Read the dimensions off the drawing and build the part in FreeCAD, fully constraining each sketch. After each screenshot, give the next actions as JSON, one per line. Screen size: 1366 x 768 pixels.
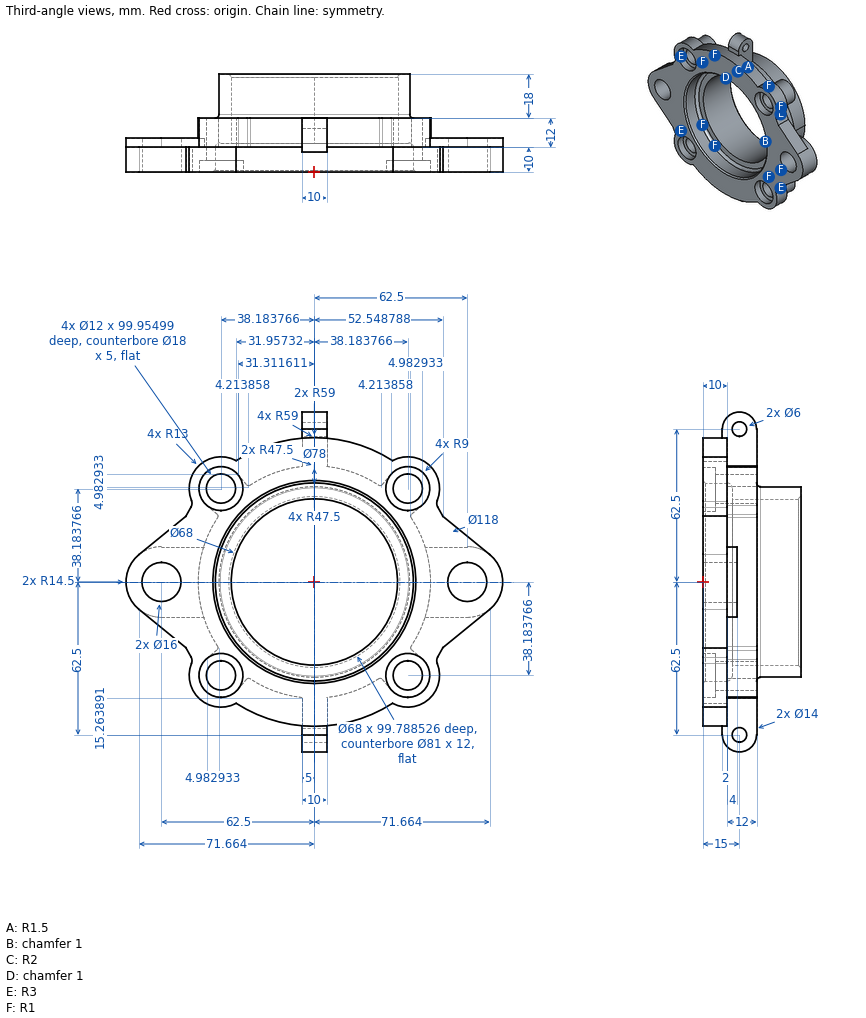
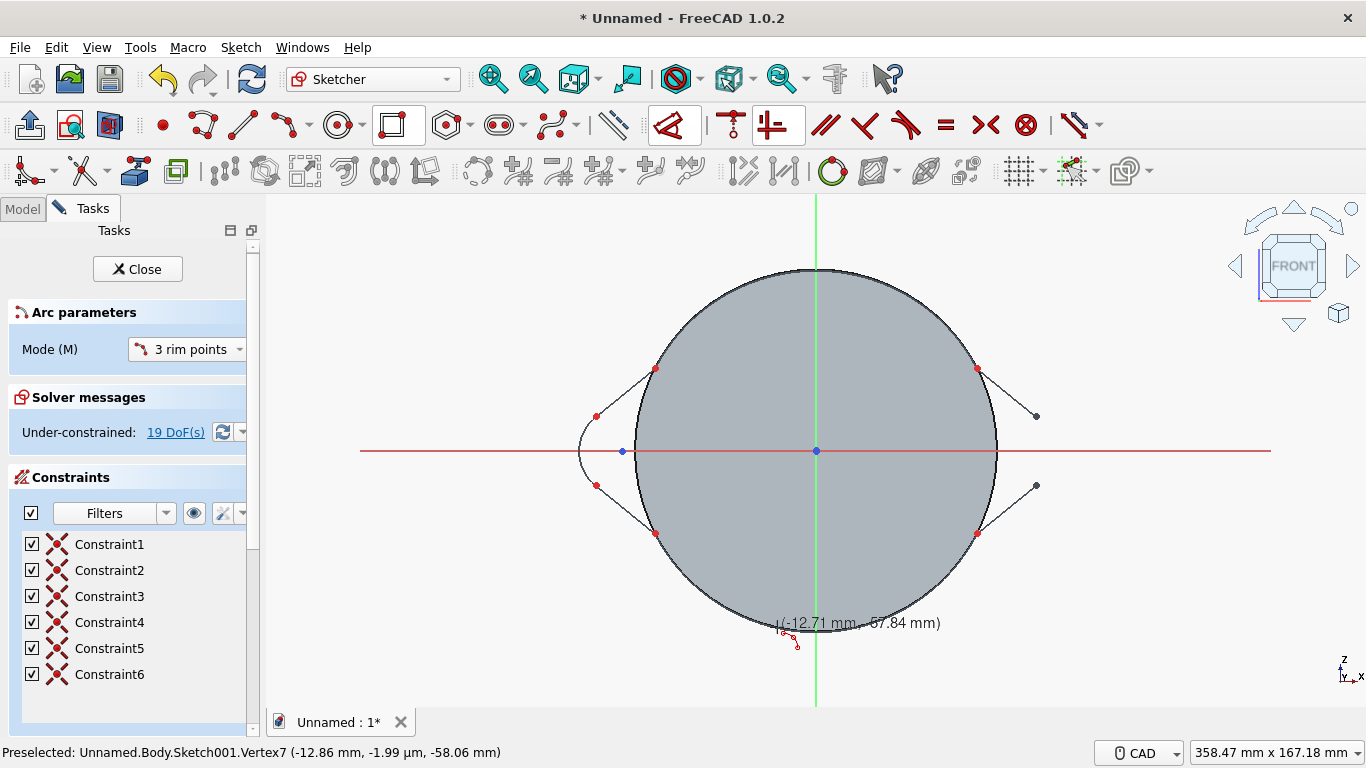
{"action": "left_click", "coordinate": [1036, 486]}
{"action": "left_click", "coordinate": [1036, 417]}
{"action": "left_click", "coordinate": [1050, 466]}
{"action": "key", "text": "Escape"}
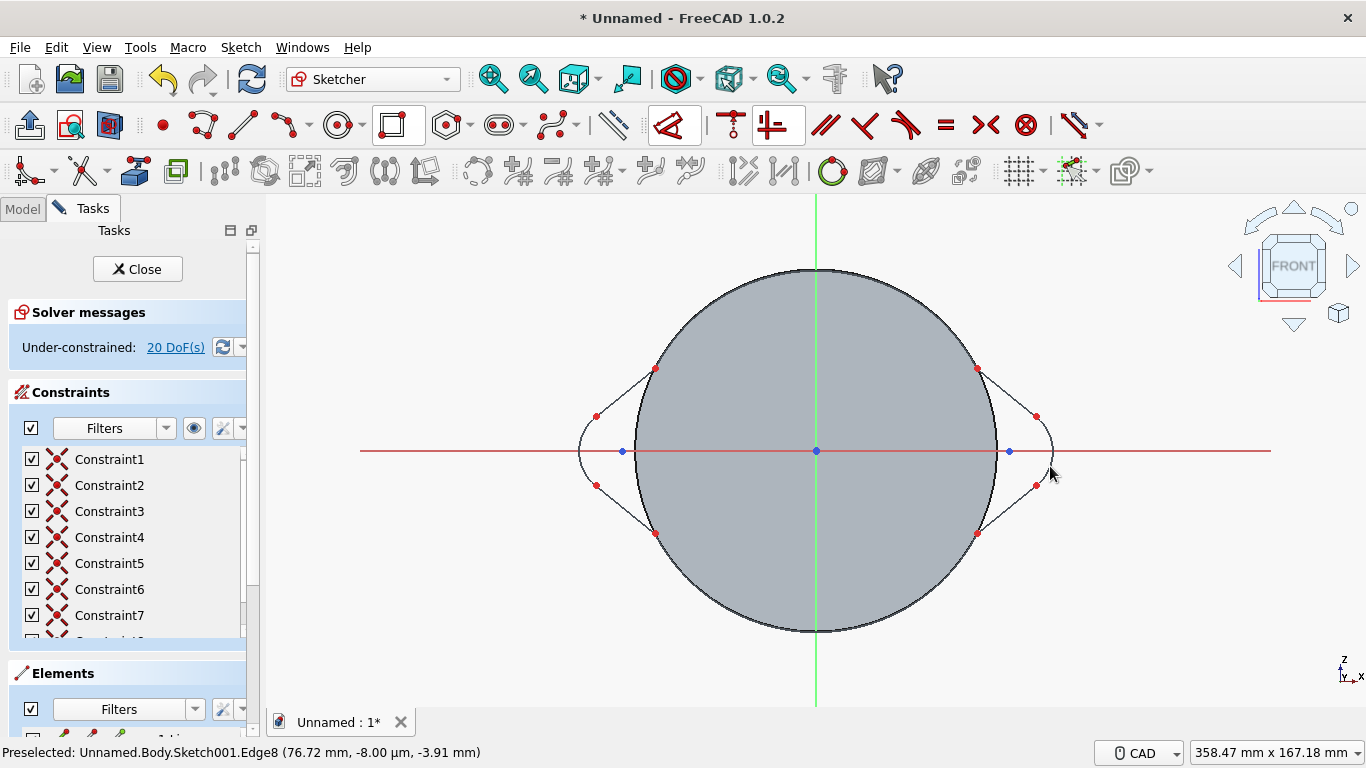
{"action": "left_click", "coordinate": [1018, 403]}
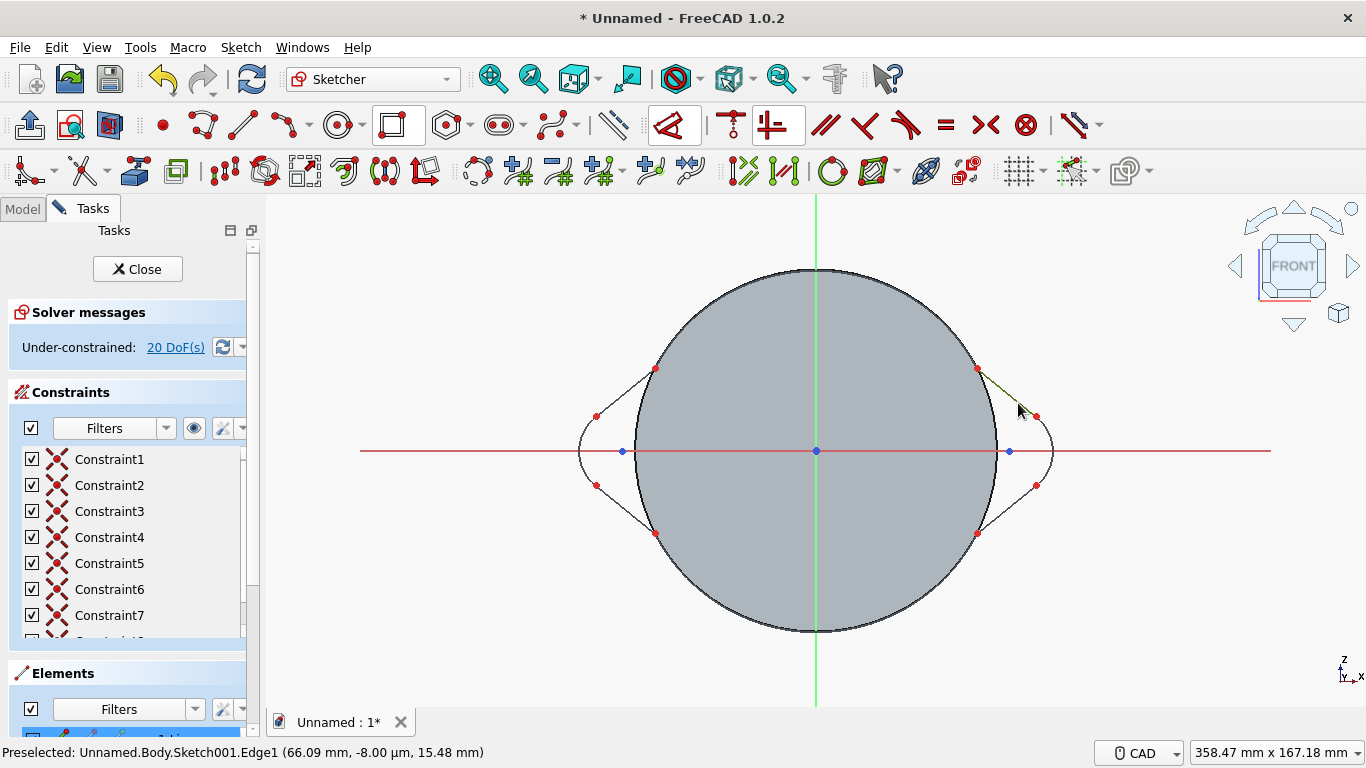
{"action": "left_click", "coordinate": [1050, 467]}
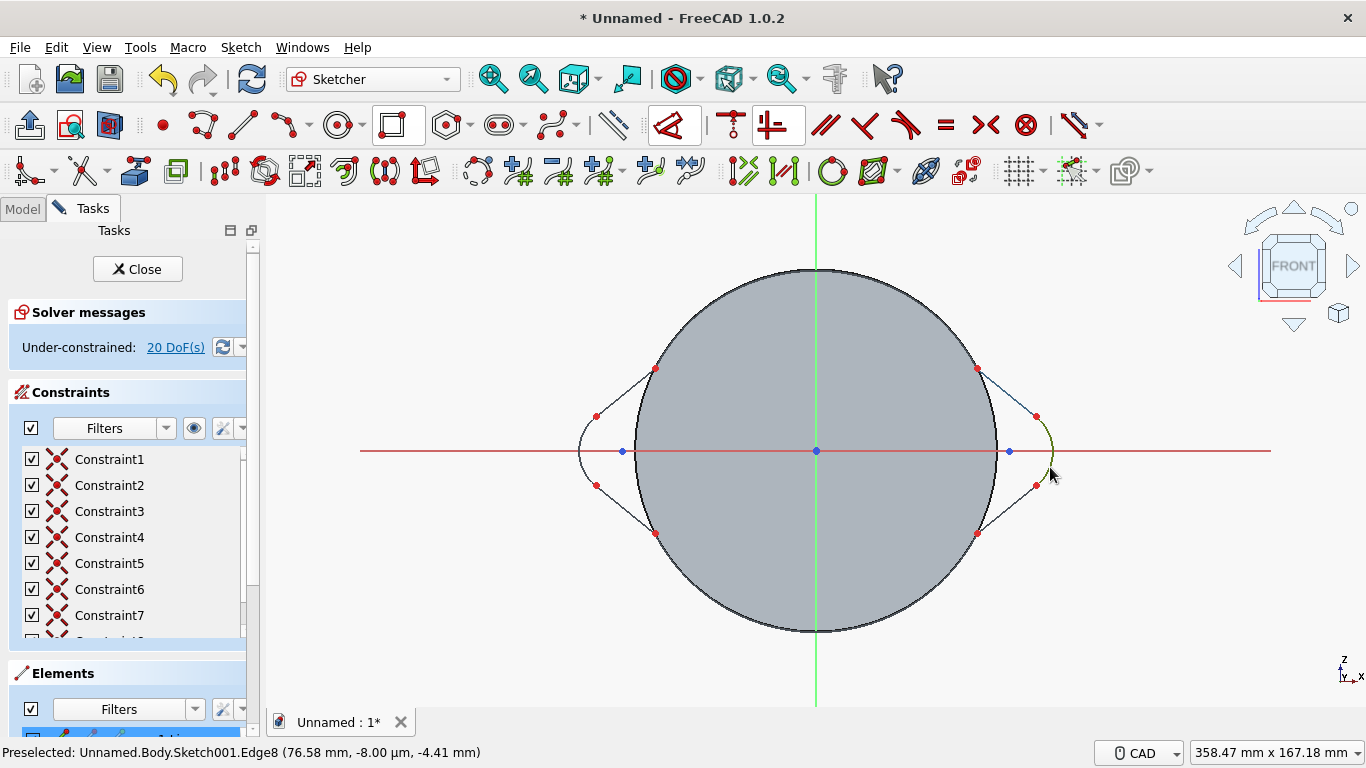
{"action": "left_click", "coordinate": [906, 126]}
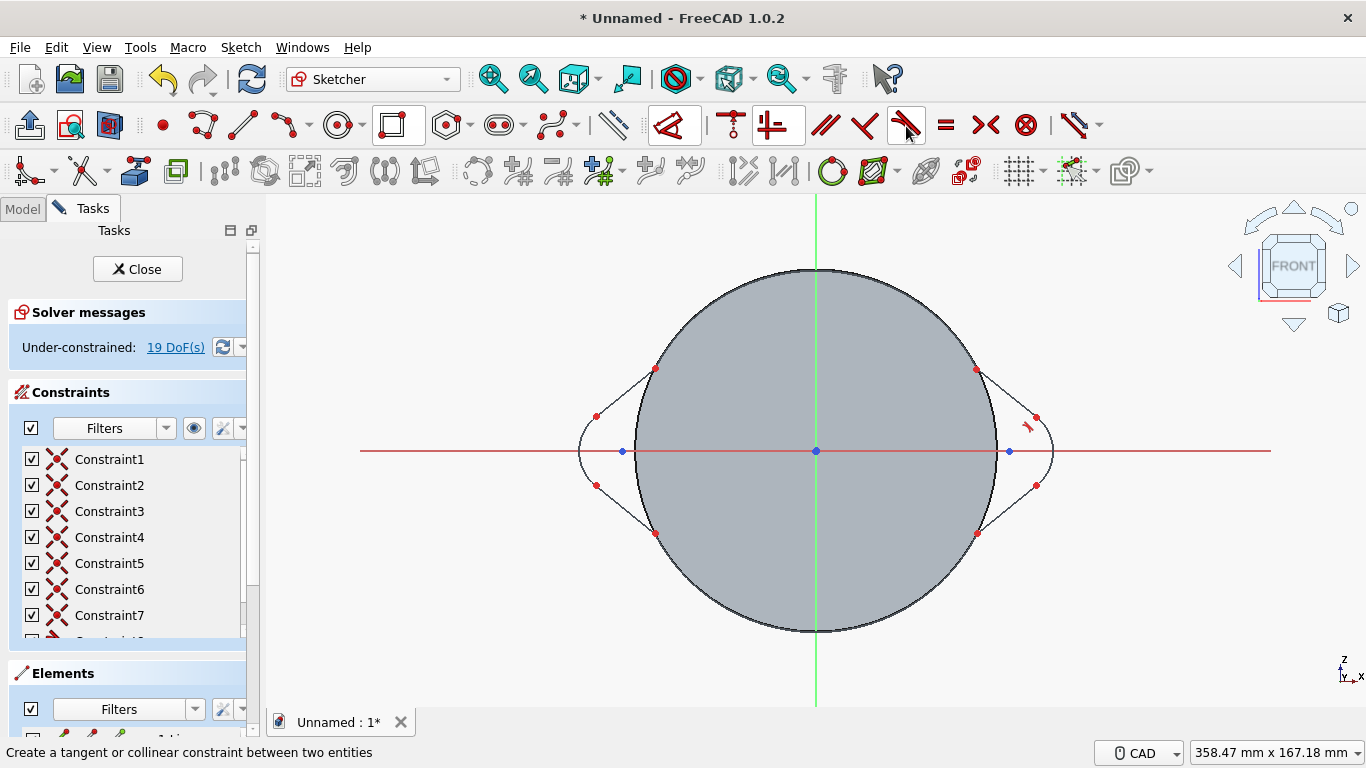
{"action": "left_click", "coordinate": [637, 383]}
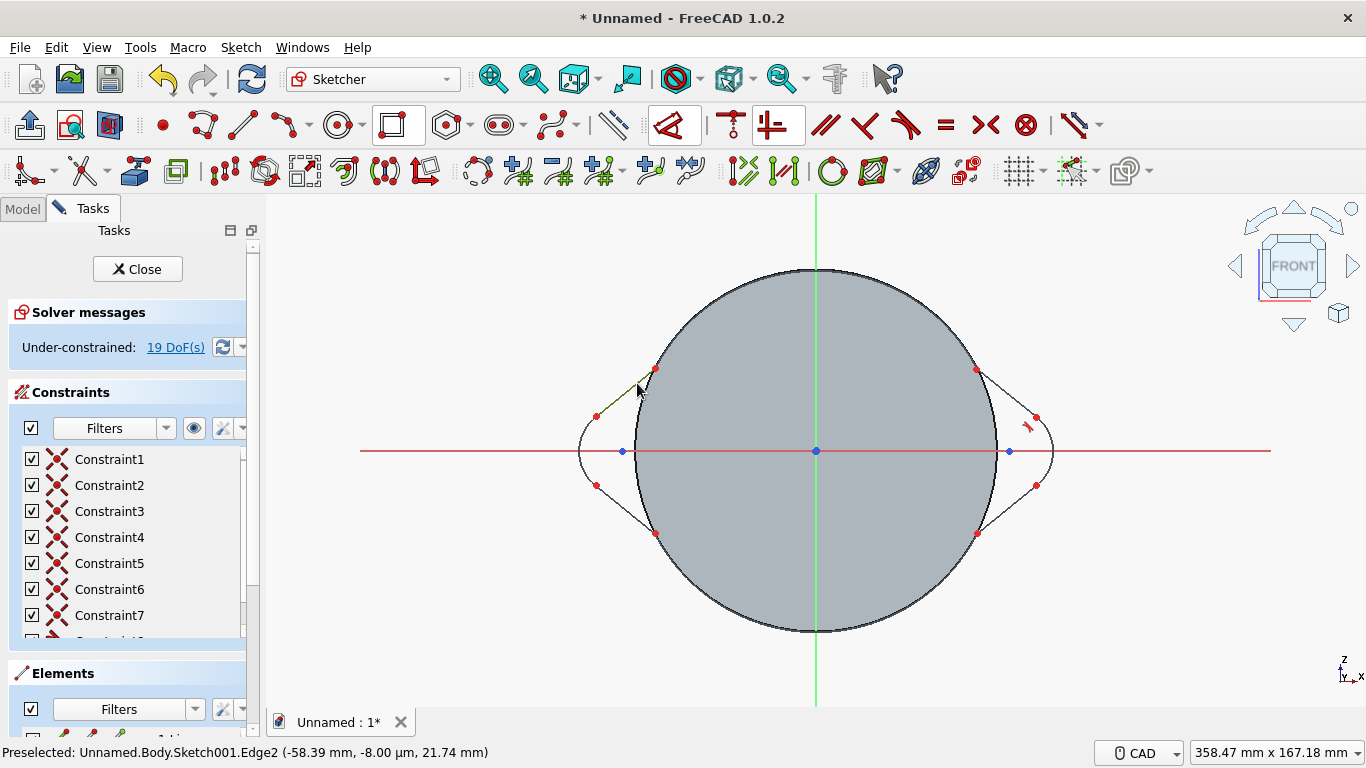
{"action": "left_click", "coordinate": [582, 436]}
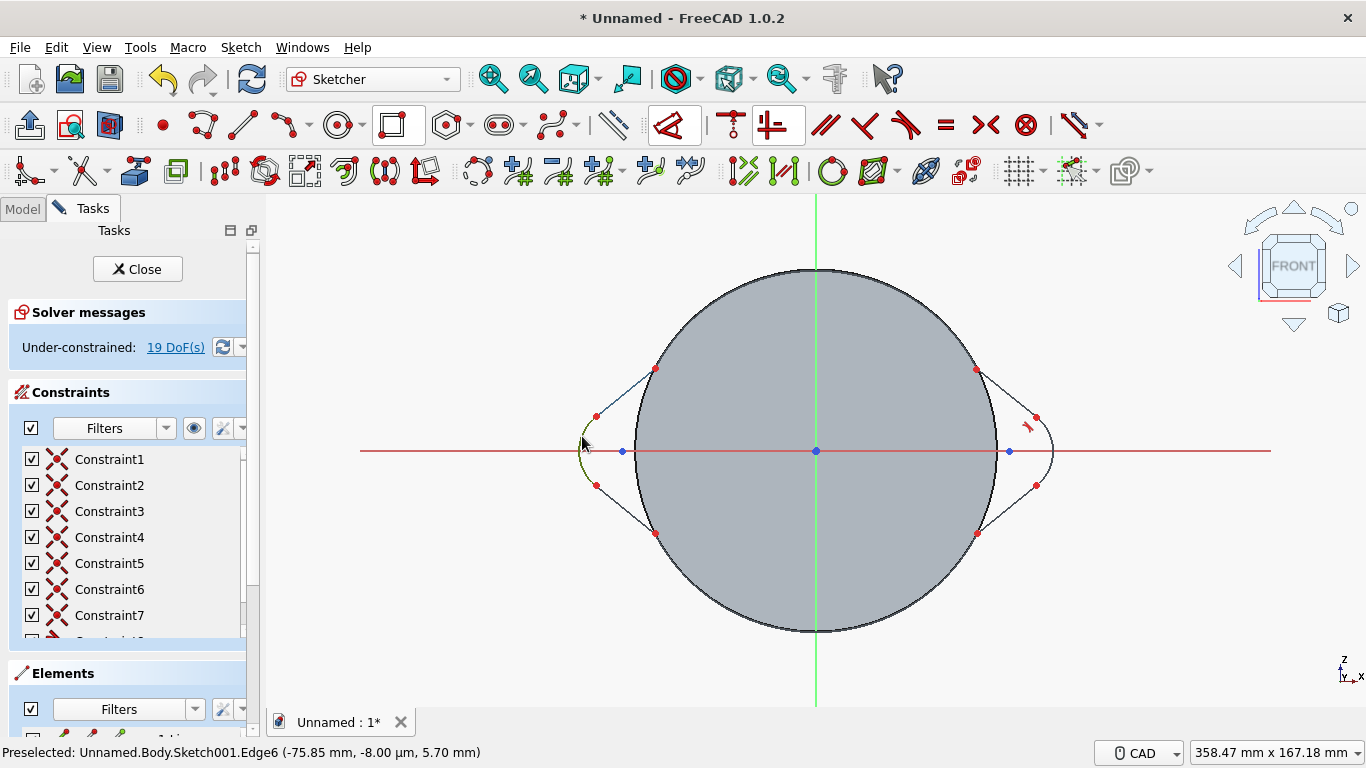
{"action": "left_click", "coordinate": [906, 126]}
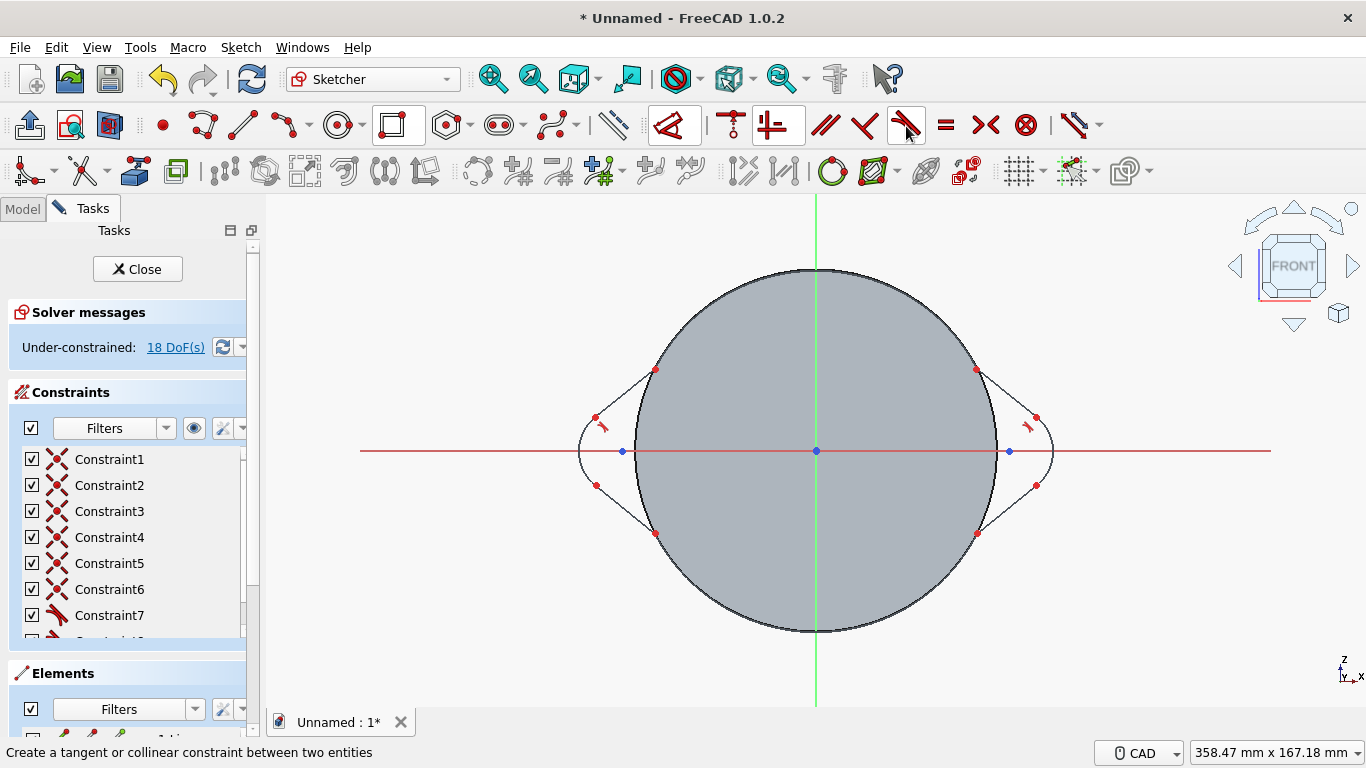
{"action": "left_click", "coordinate": [614, 500]}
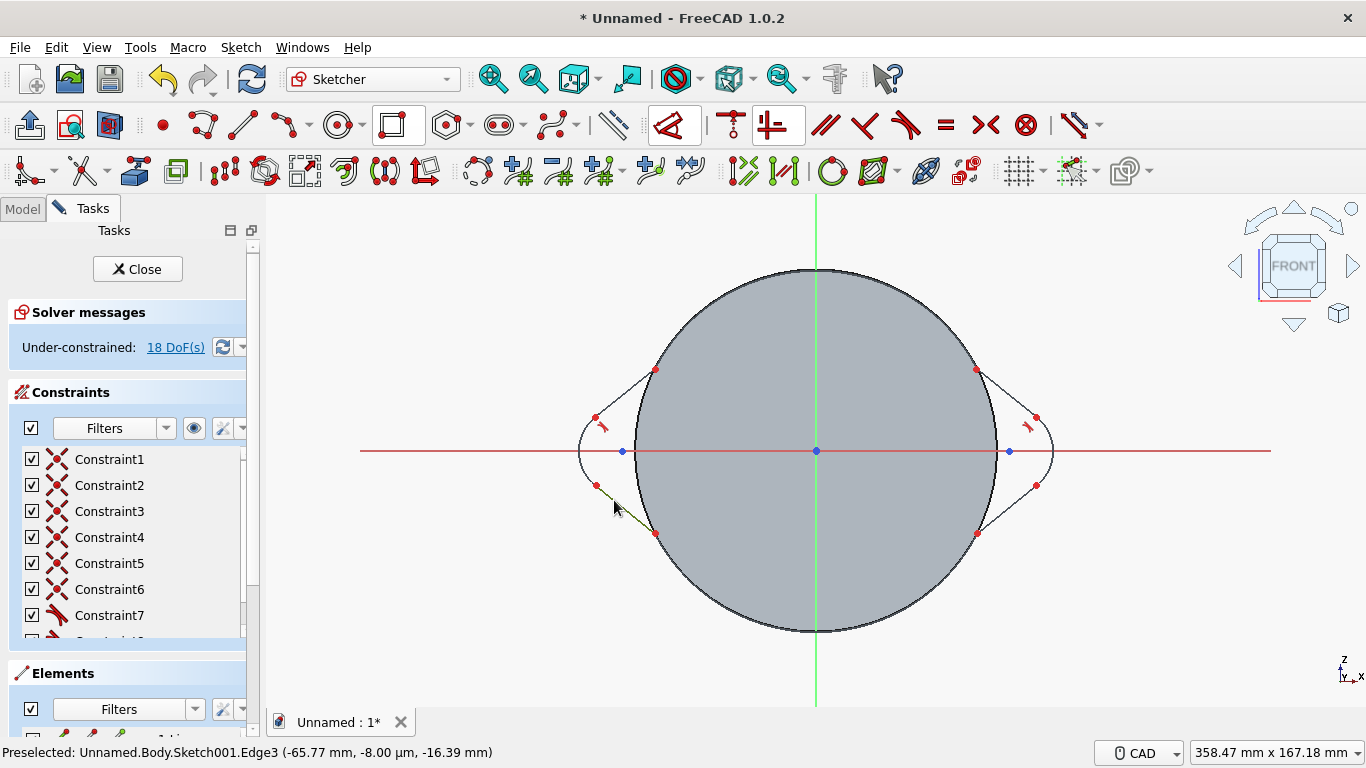
{"action": "left_click", "coordinate": [582, 436]}